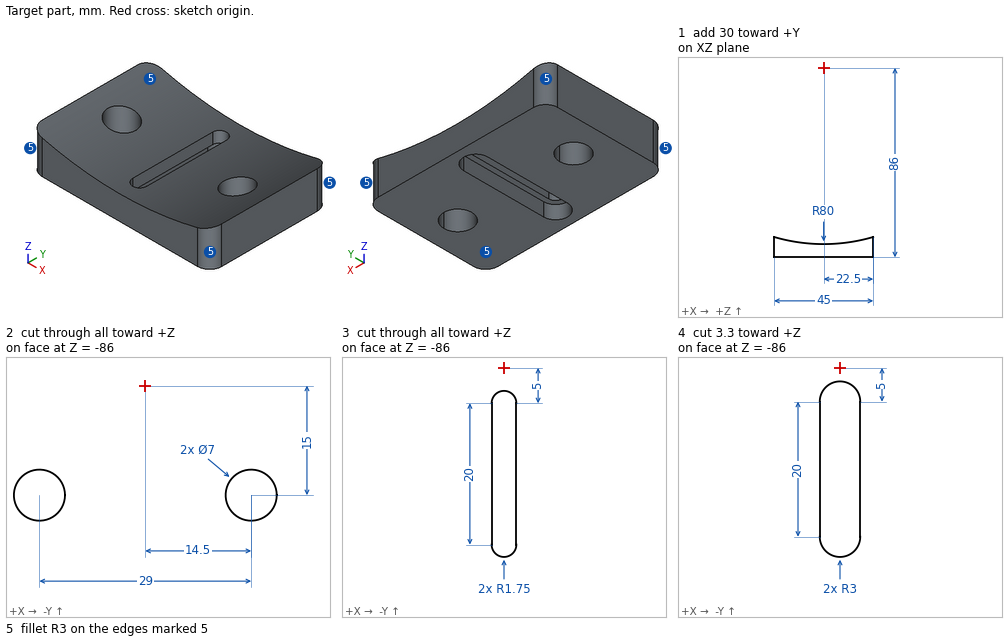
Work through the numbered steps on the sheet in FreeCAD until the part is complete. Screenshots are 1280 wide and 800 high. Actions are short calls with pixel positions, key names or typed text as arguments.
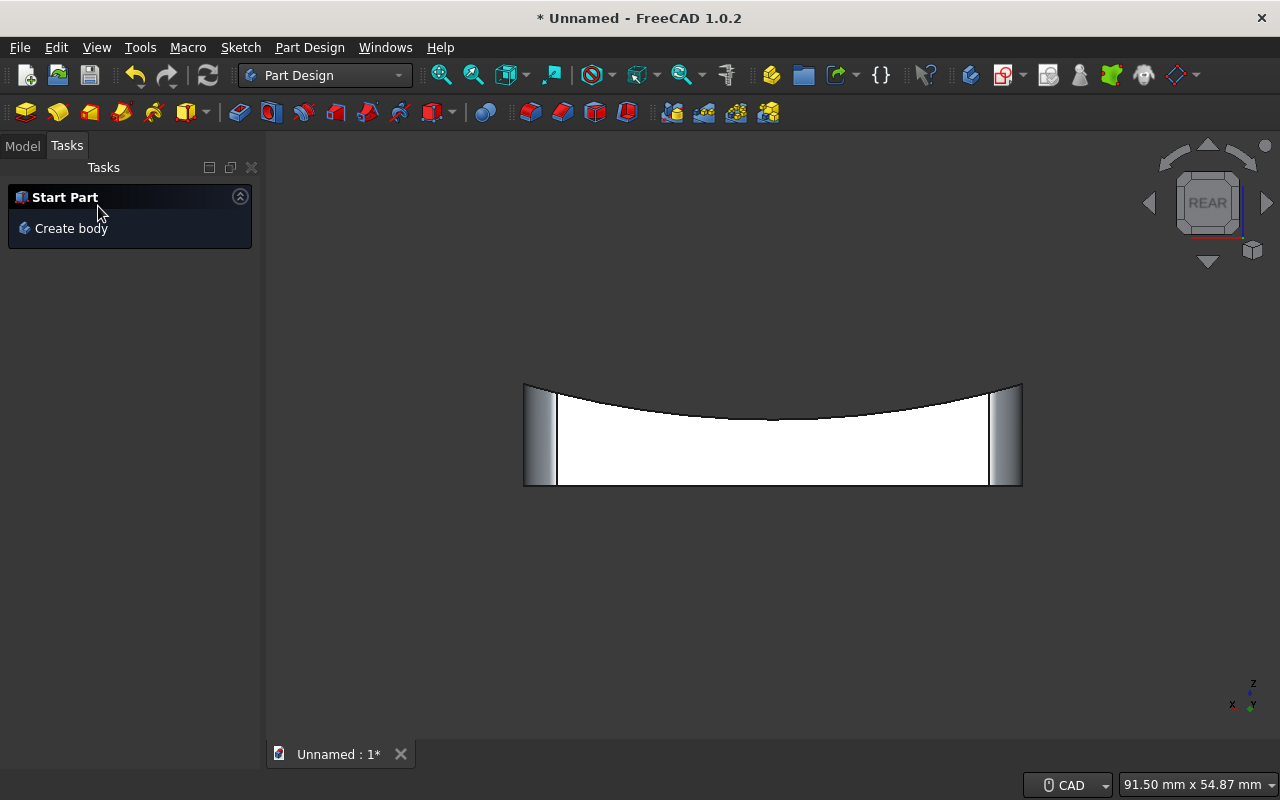
key(0)